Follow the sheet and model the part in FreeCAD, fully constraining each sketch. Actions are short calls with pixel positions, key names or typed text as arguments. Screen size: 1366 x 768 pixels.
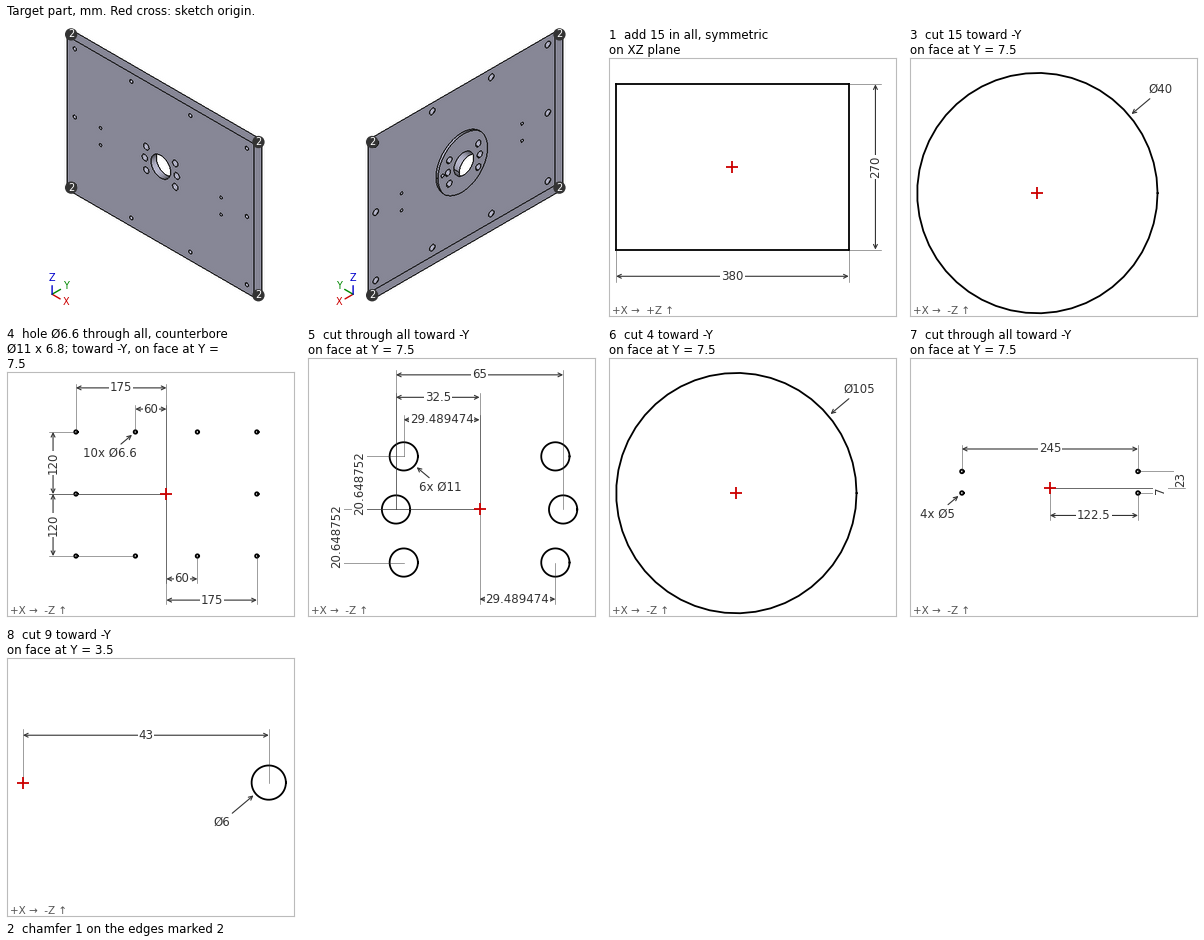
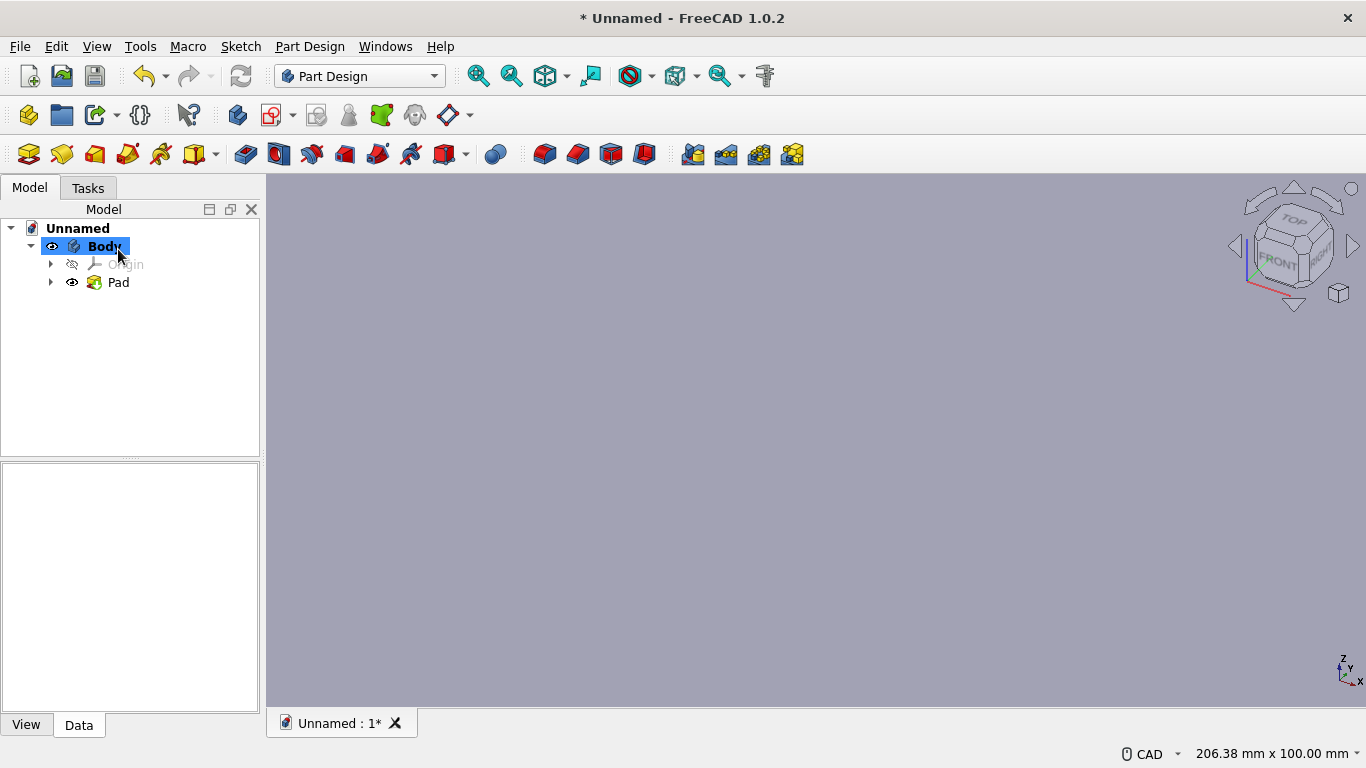
click(479, 76)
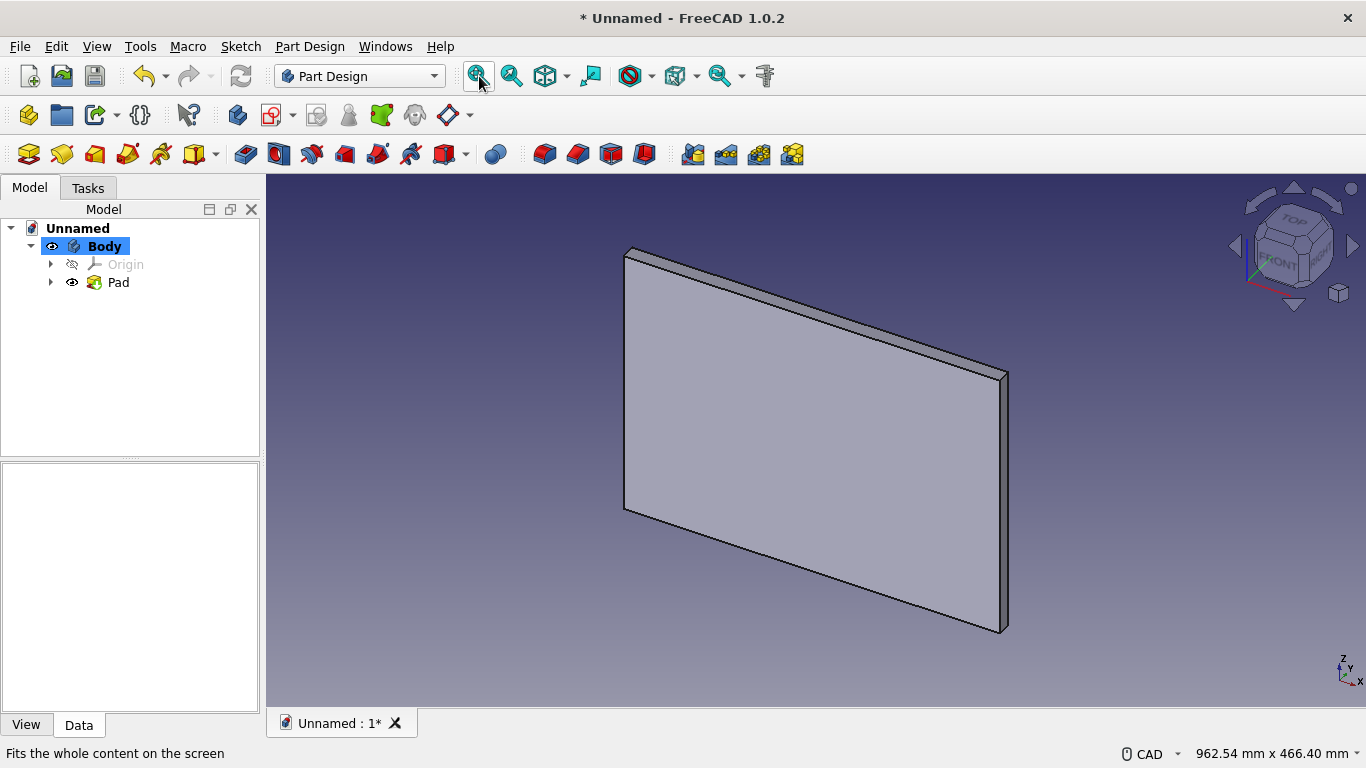
click(1005, 375)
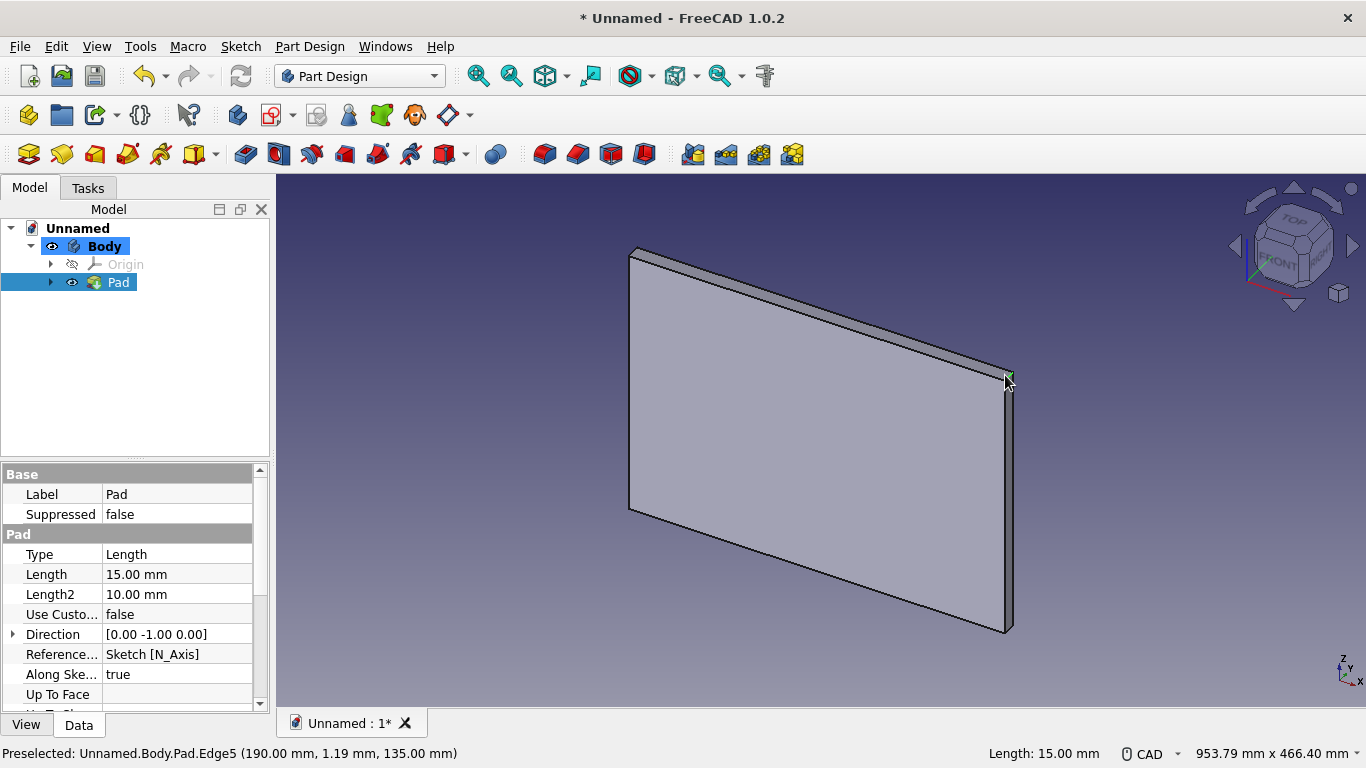
scroll(633, 251, up, 5)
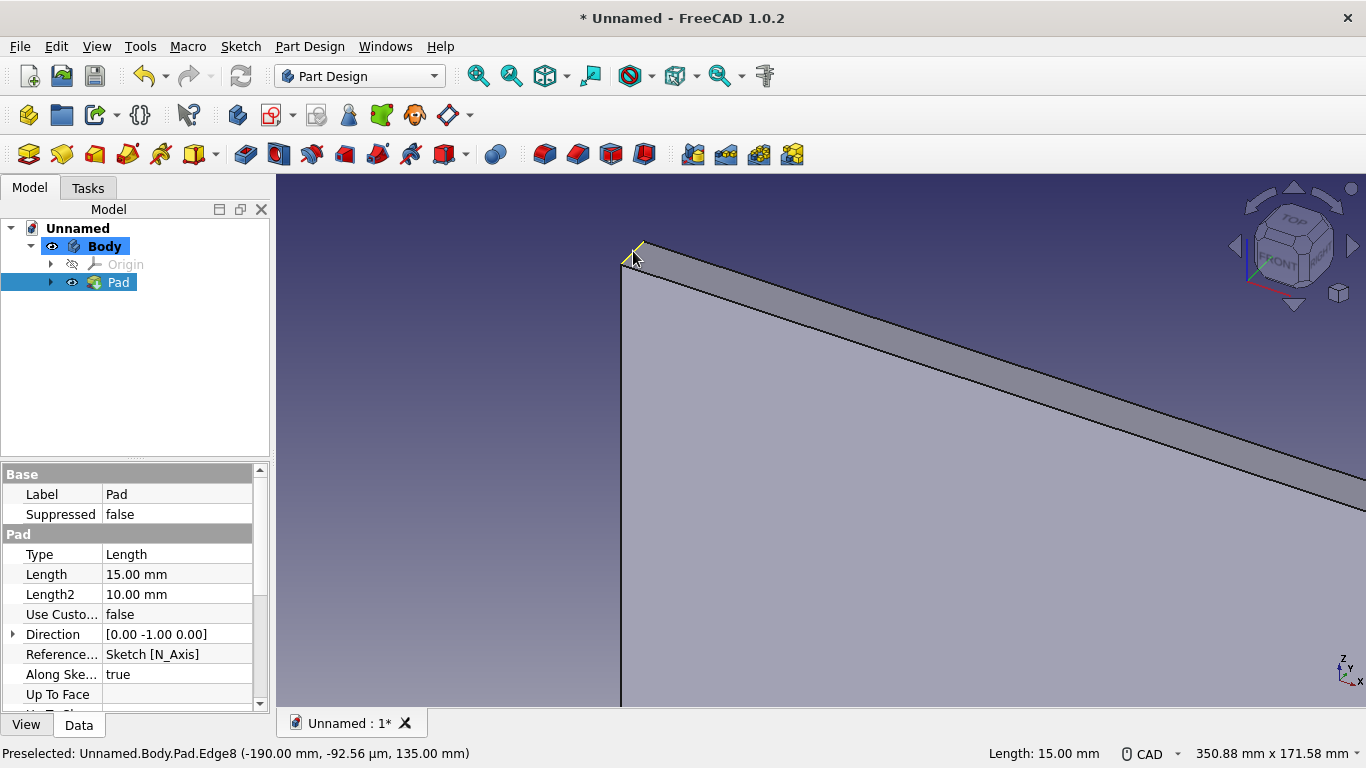
click(479, 76)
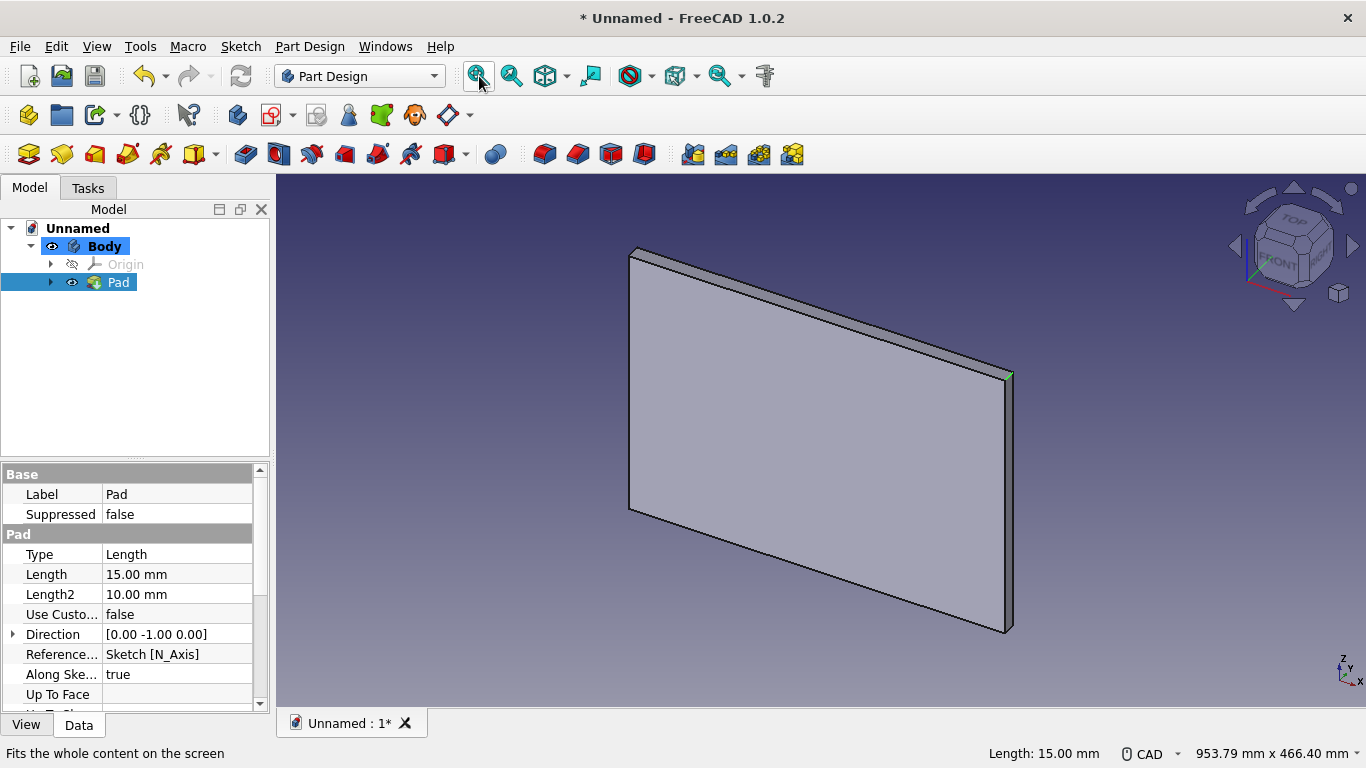
key(0)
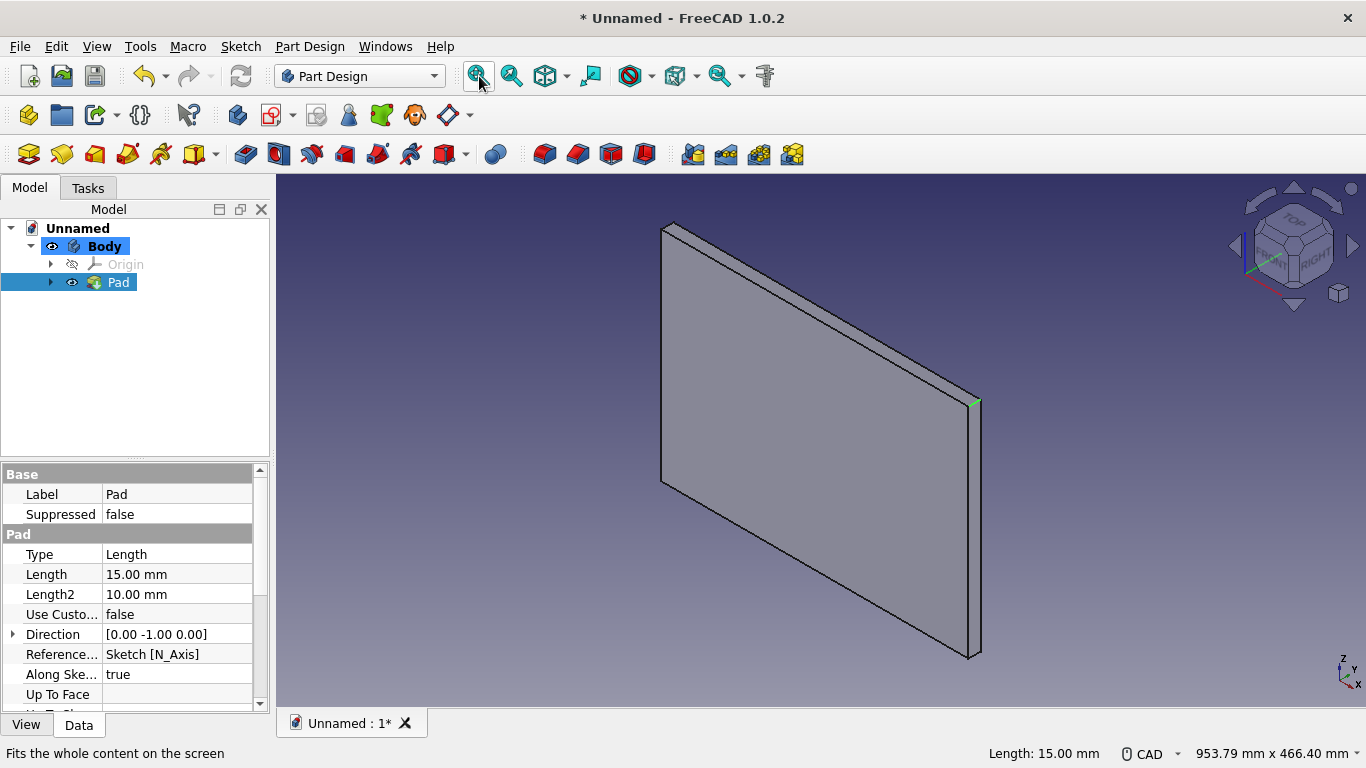
scroll(667, 225, up, 5)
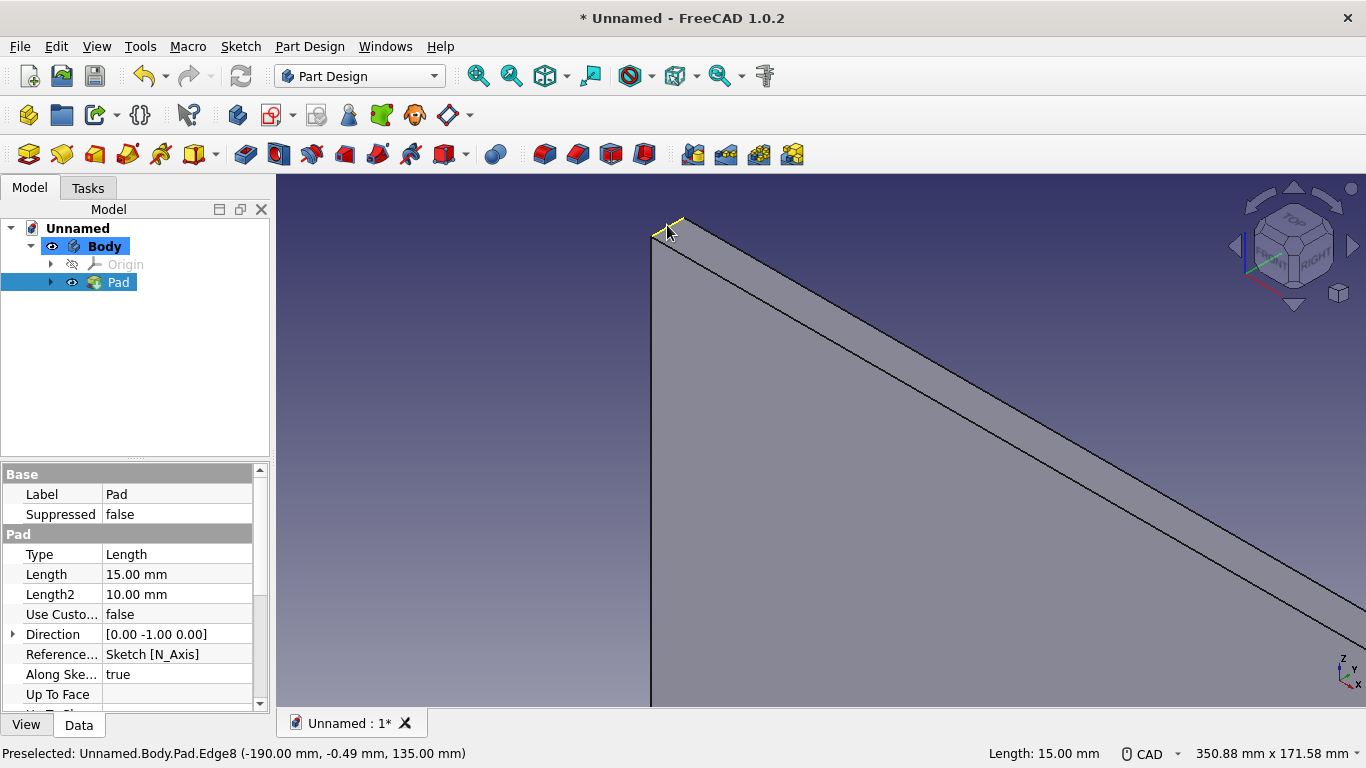
click(479, 76)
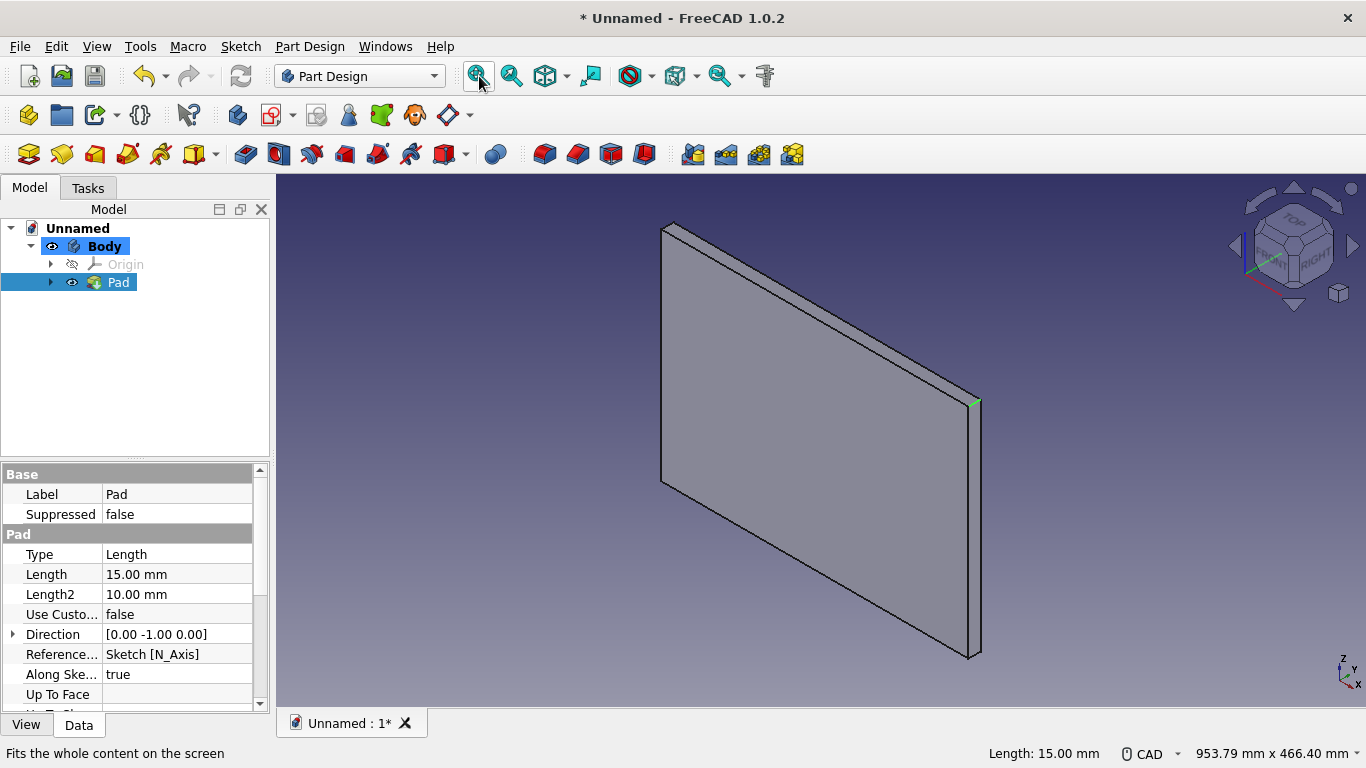
key(2)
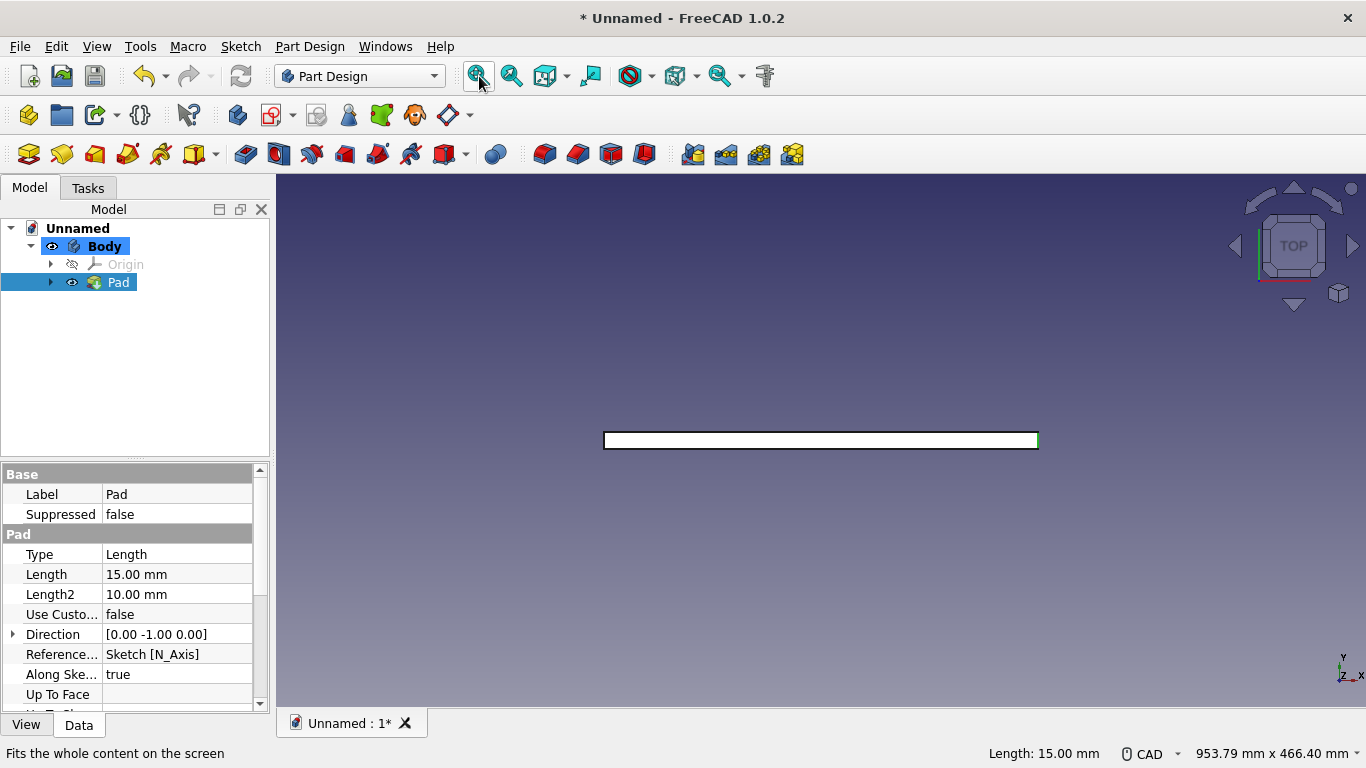
click(479, 76)